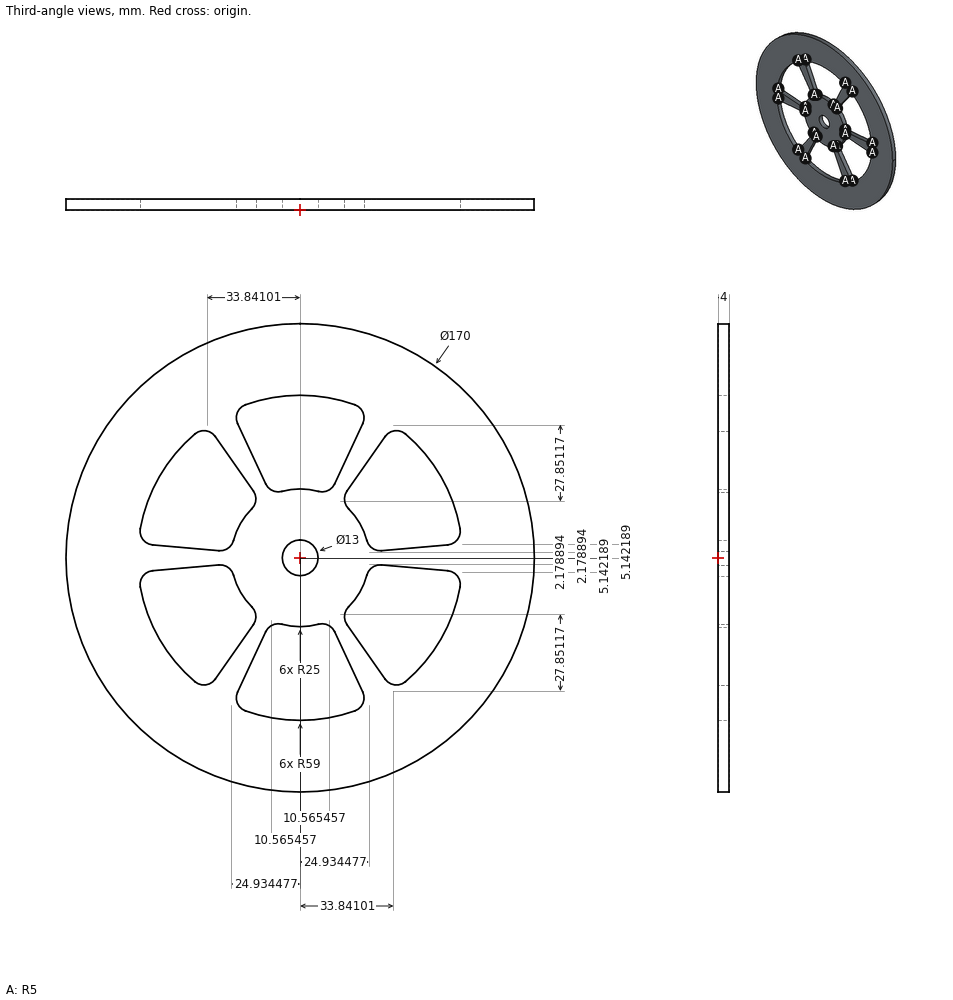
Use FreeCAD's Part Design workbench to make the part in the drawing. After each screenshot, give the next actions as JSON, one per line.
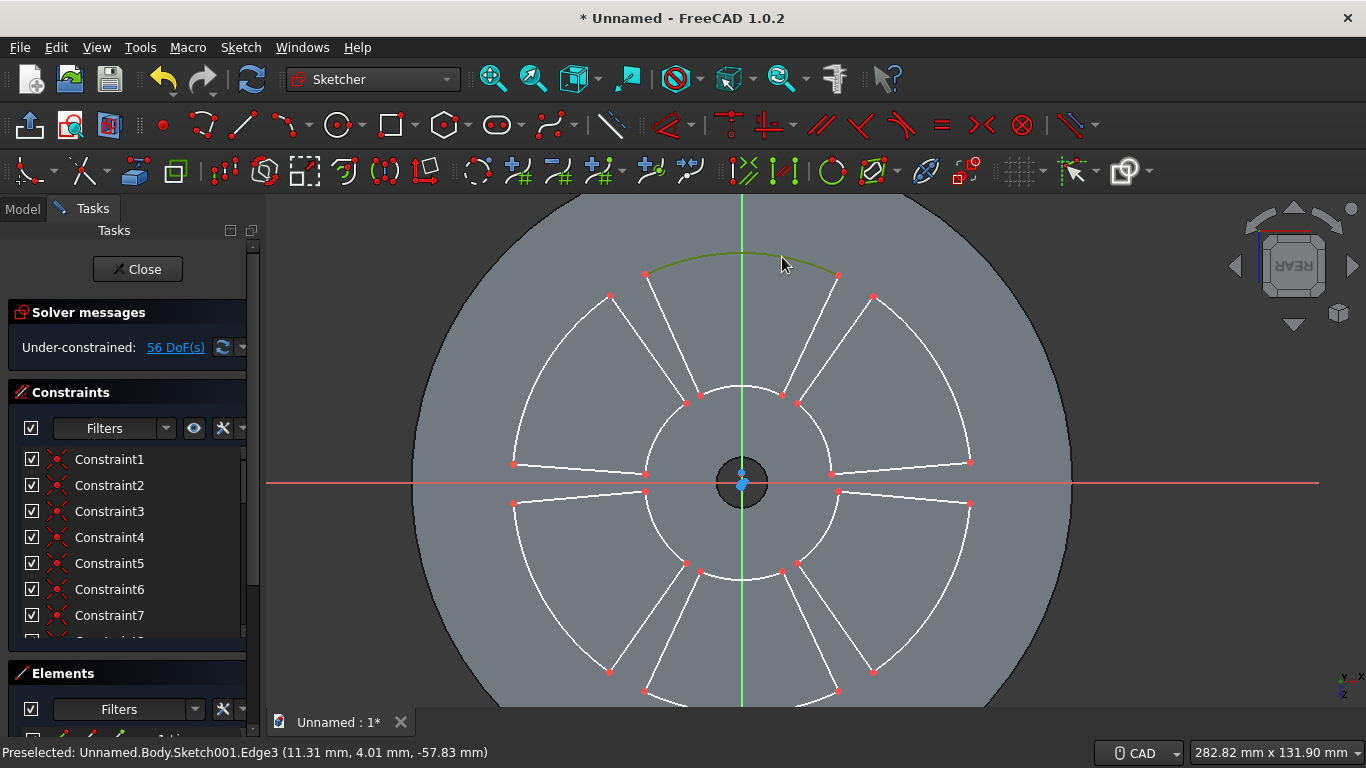
{"action": "left_click", "coordinate": [957, 405]}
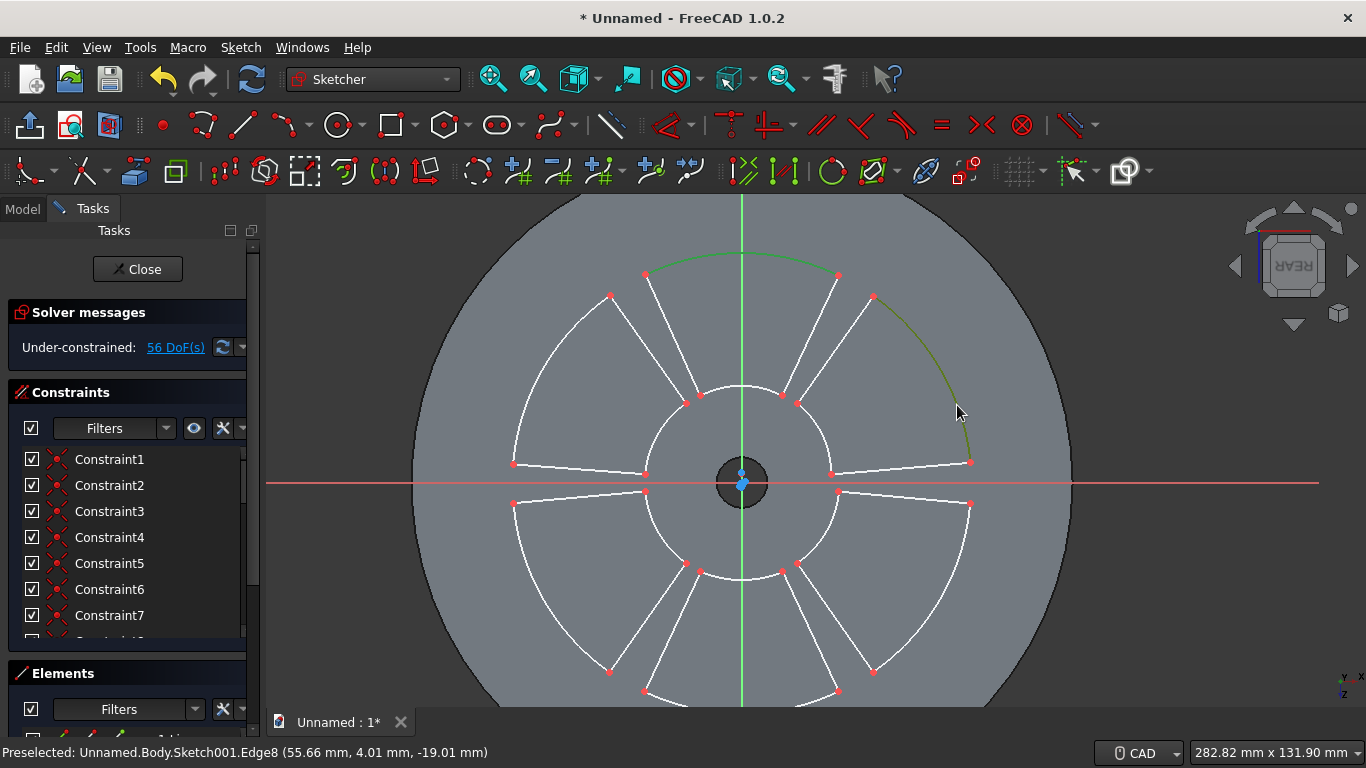
{"action": "left_click", "coordinate": [730, 126]}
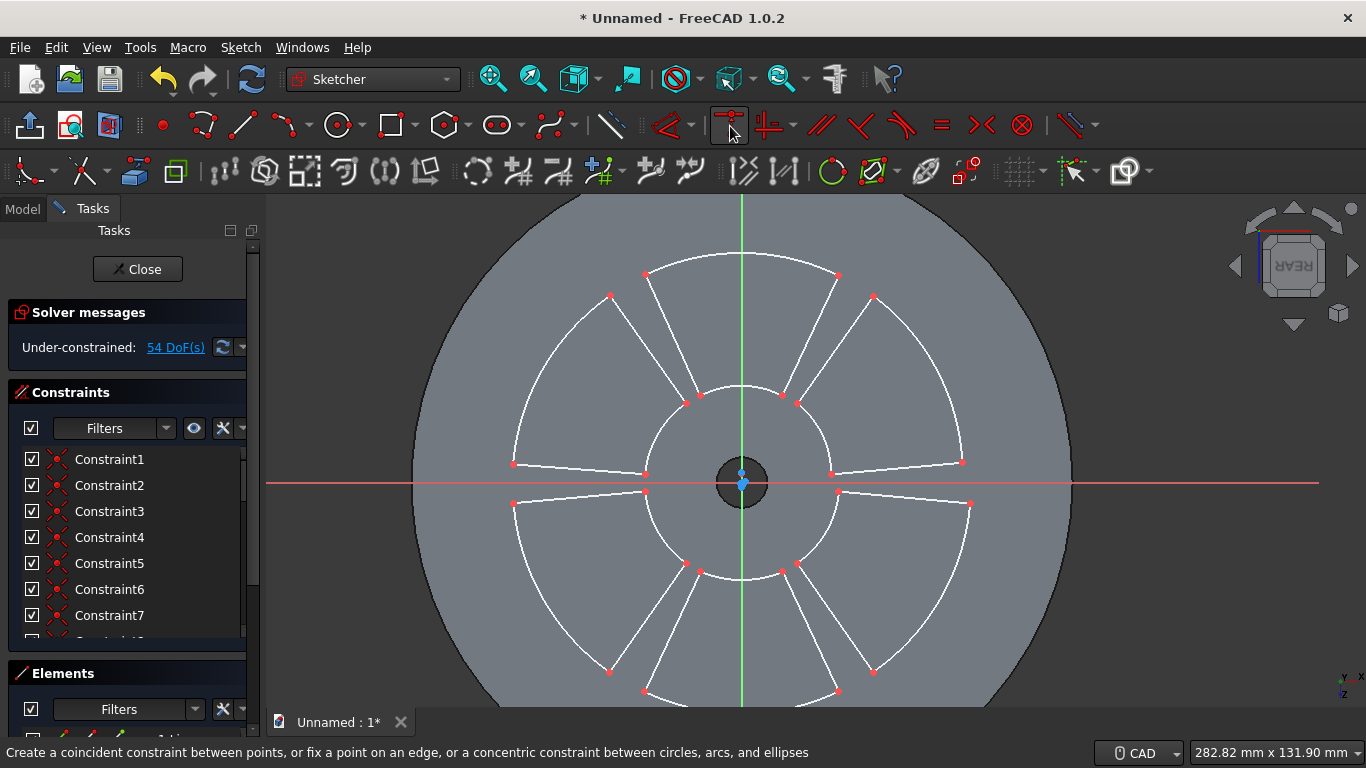
{"action": "left_click", "coordinate": [782, 257]}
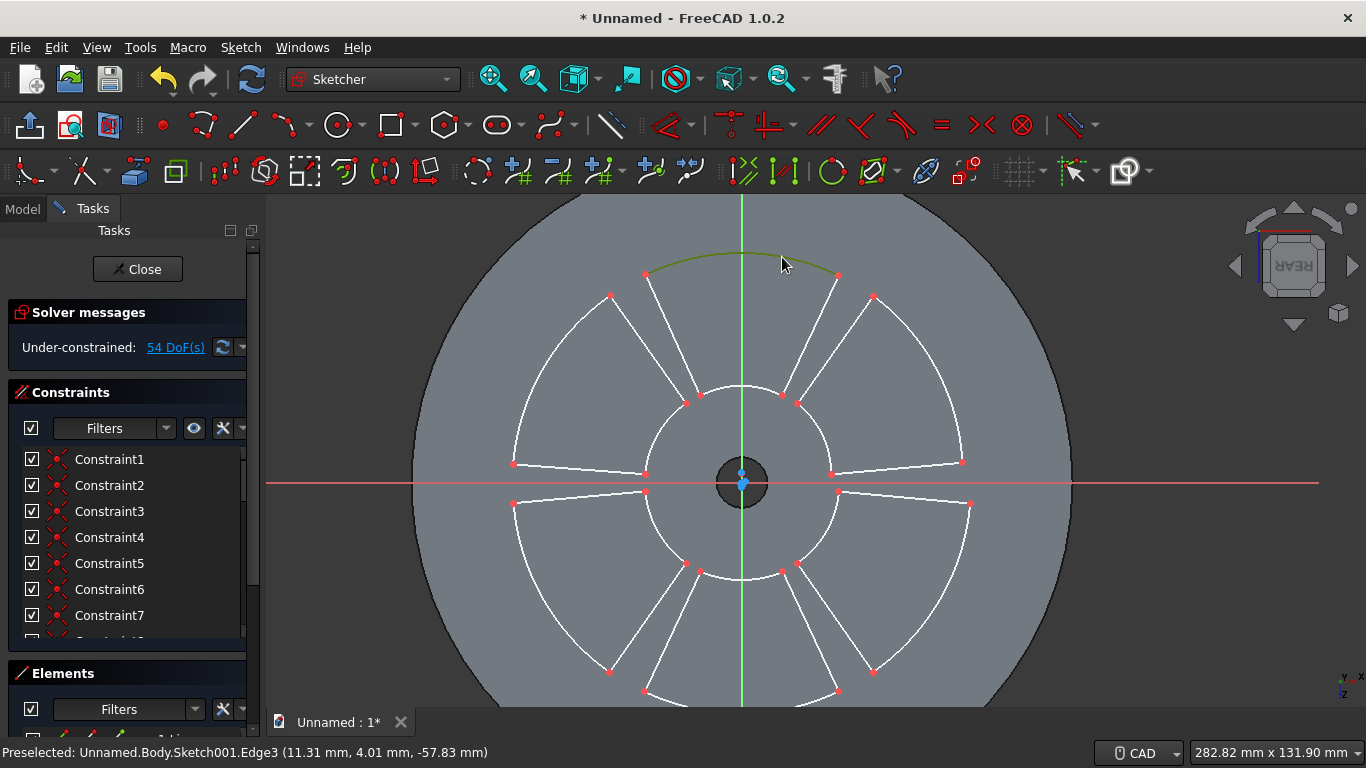
{"action": "left_click", "coordinate": [816, 546]}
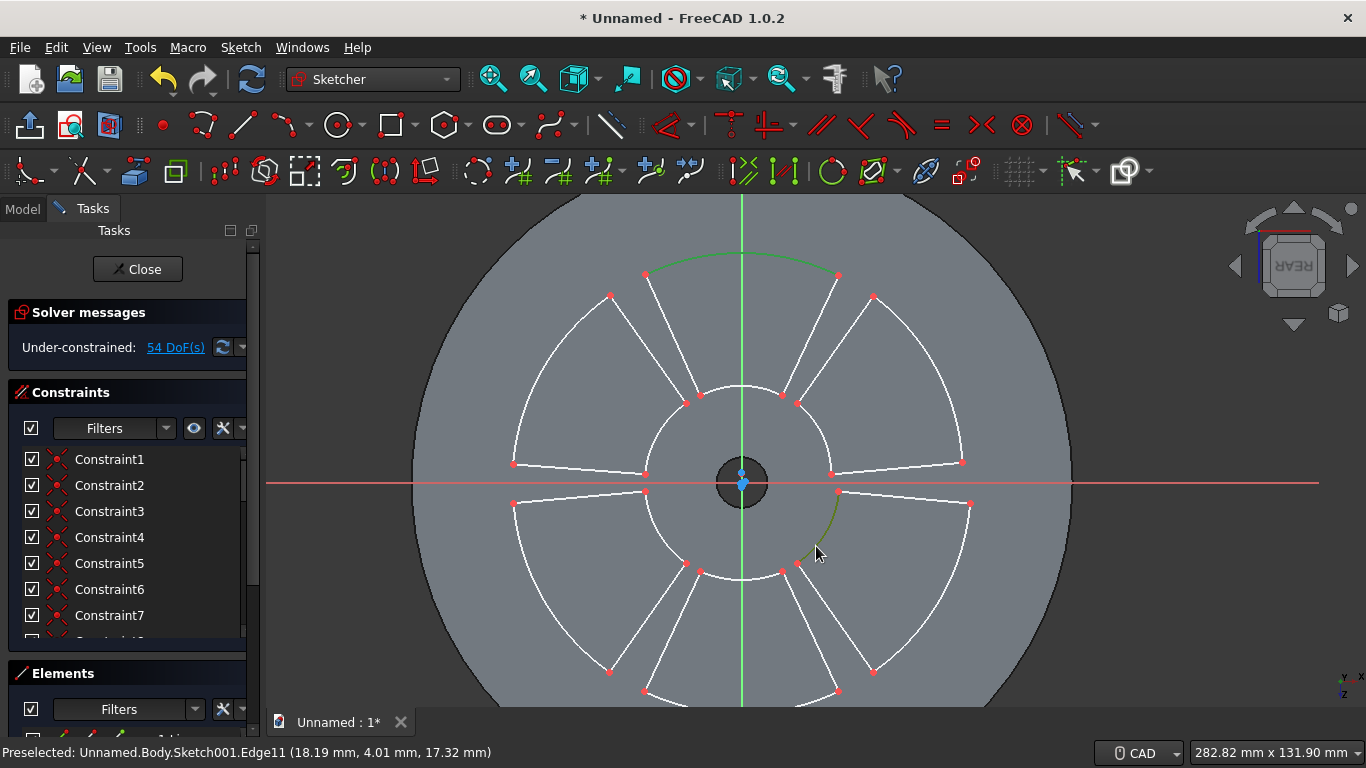
{"action": "left_click", "coordinate": [730, 126]}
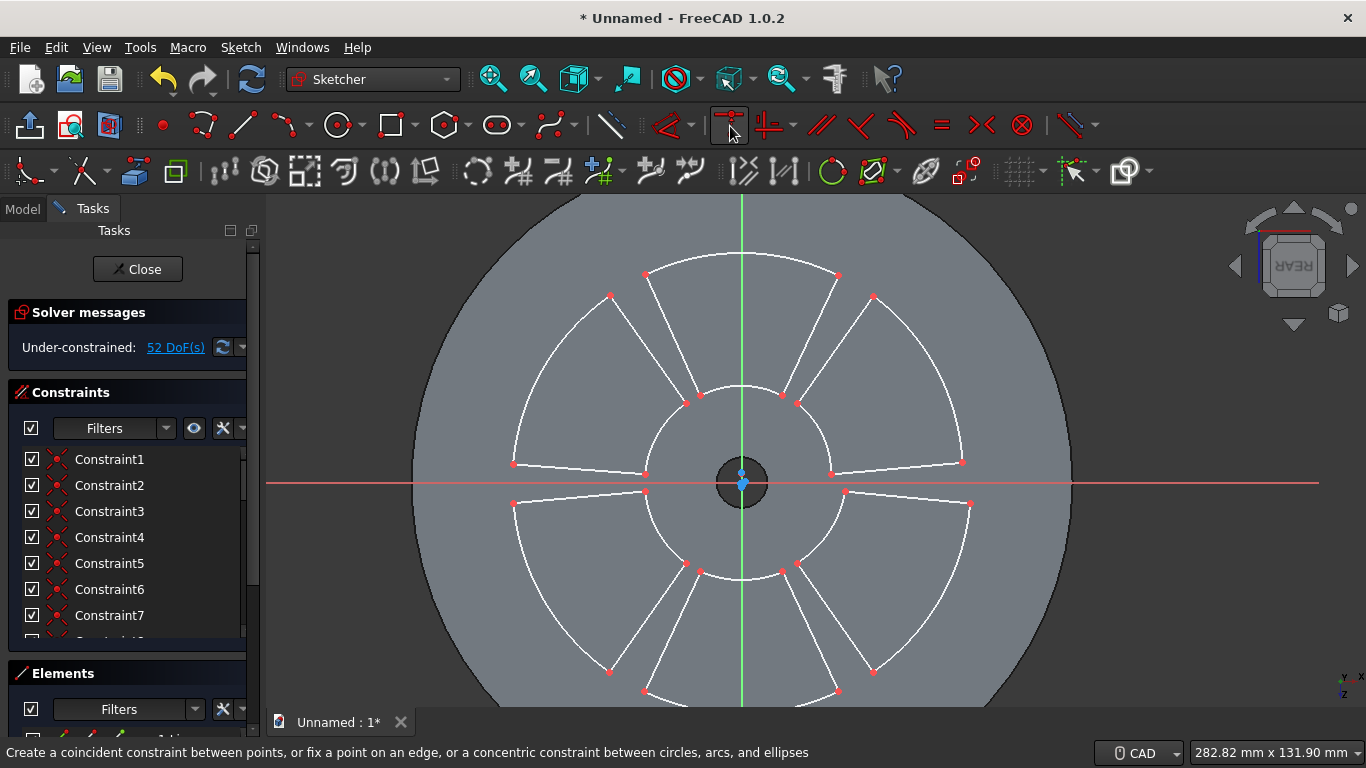
{"action": "left_click", "coordinate": [782, 257]}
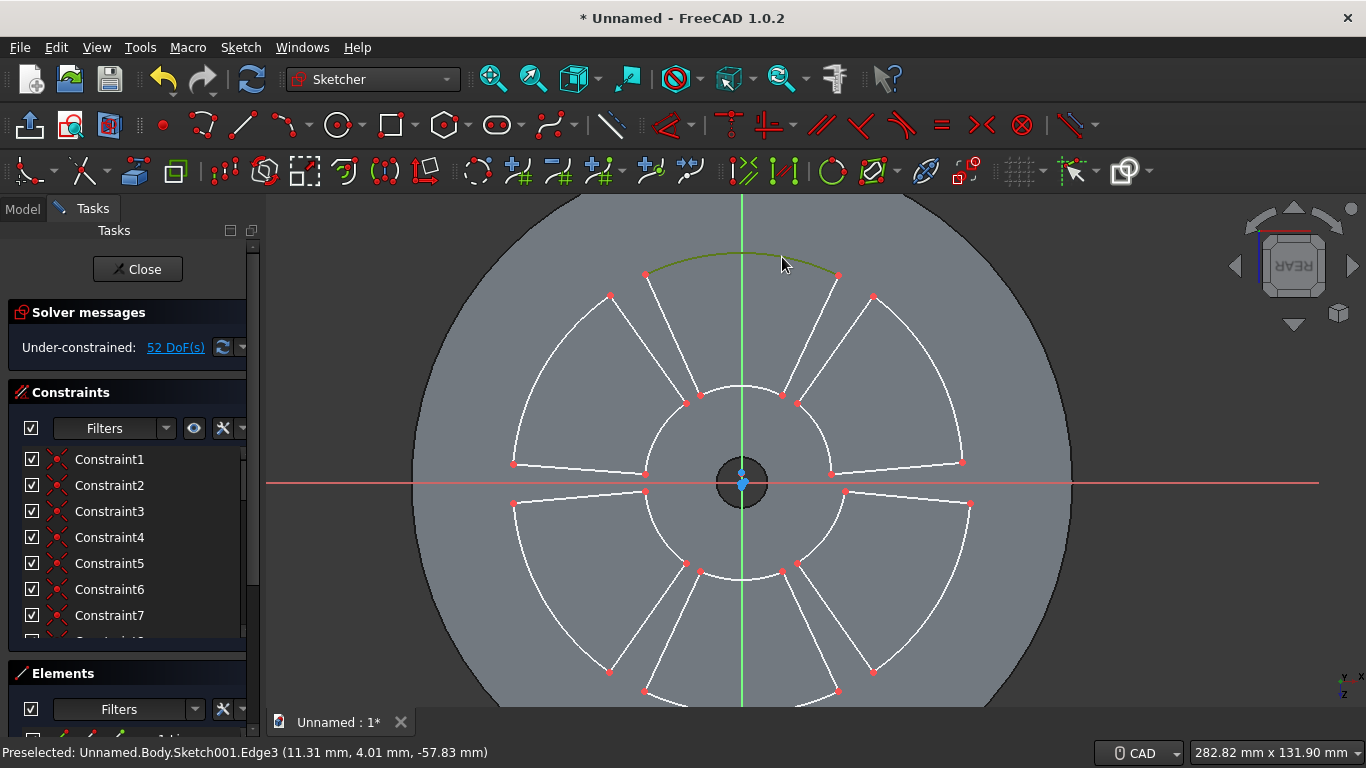
{"action": "left_click", "coordinate": [918, 631]}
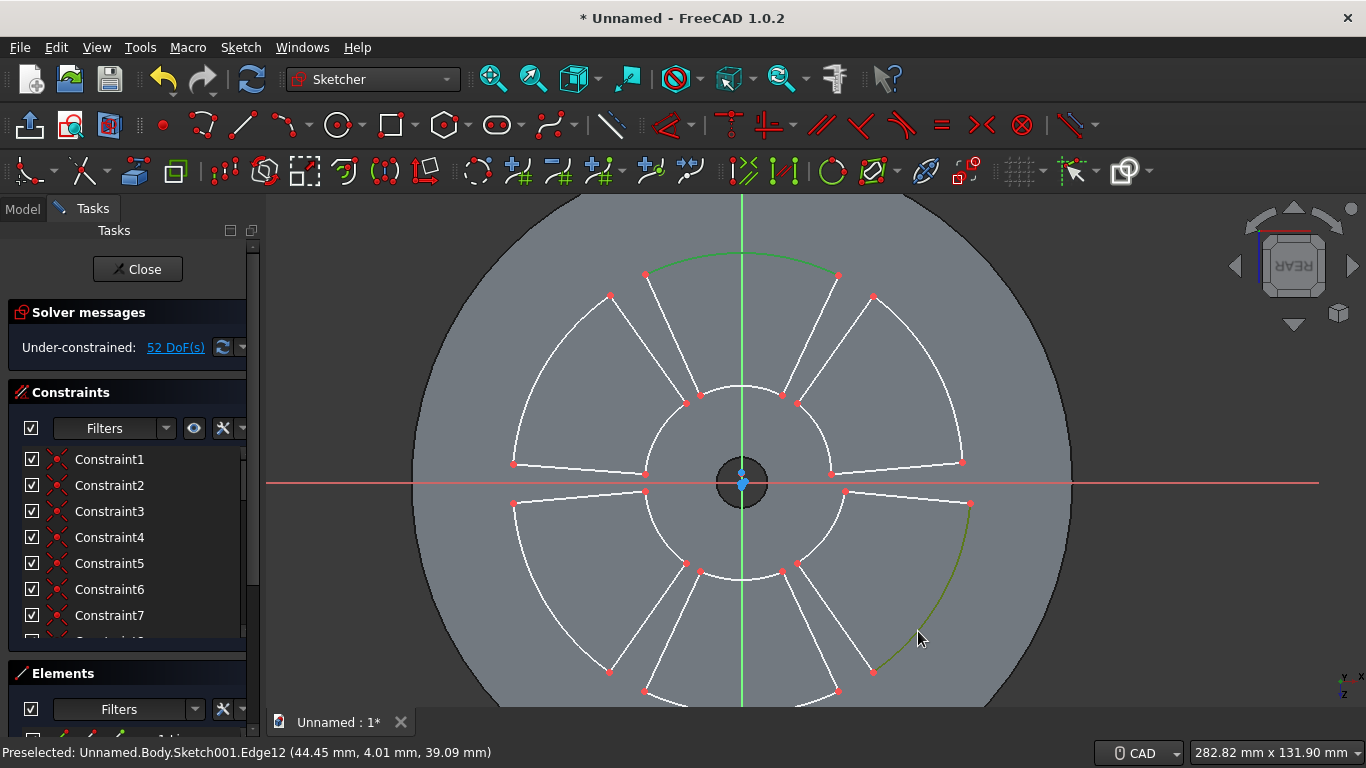
{"action": "left_click", "coordinate": [730, 126]}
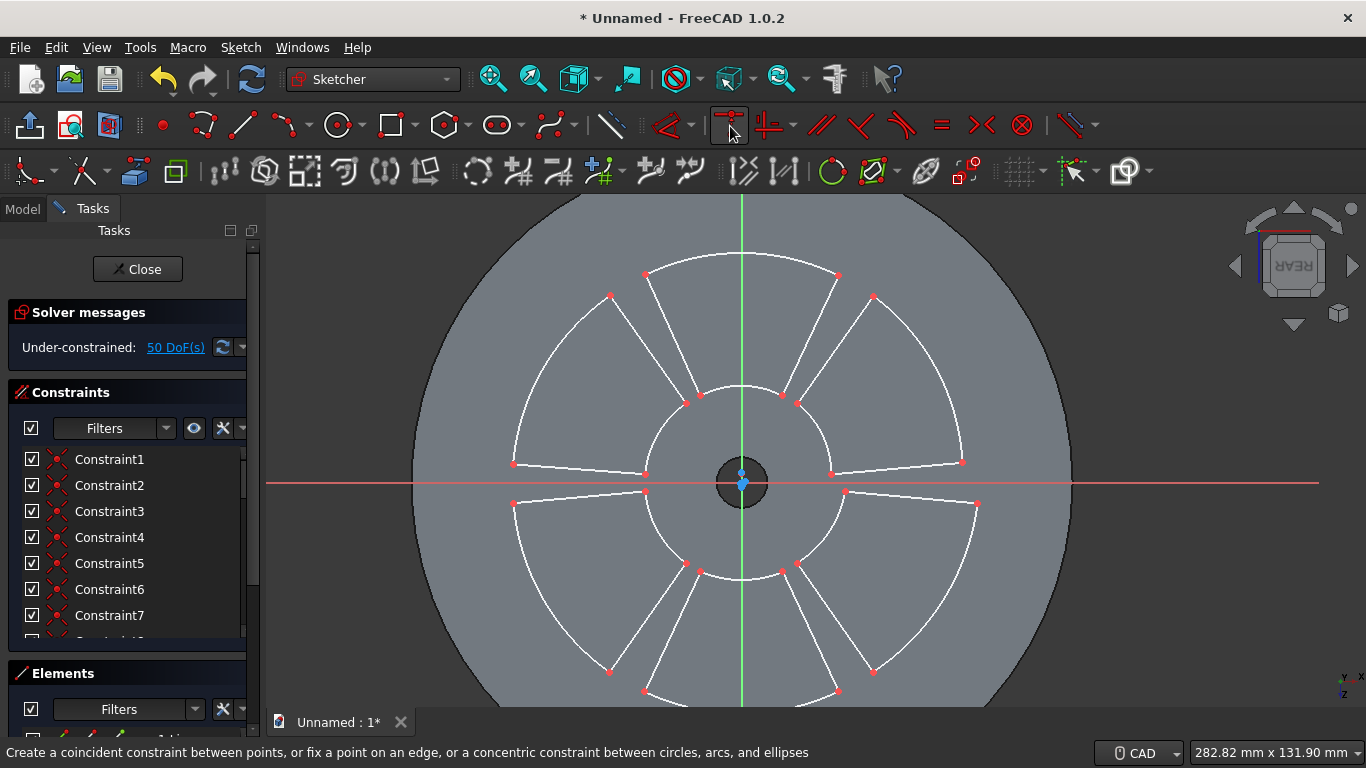
{"action": "left_click", "coordinate": [782, 257]}